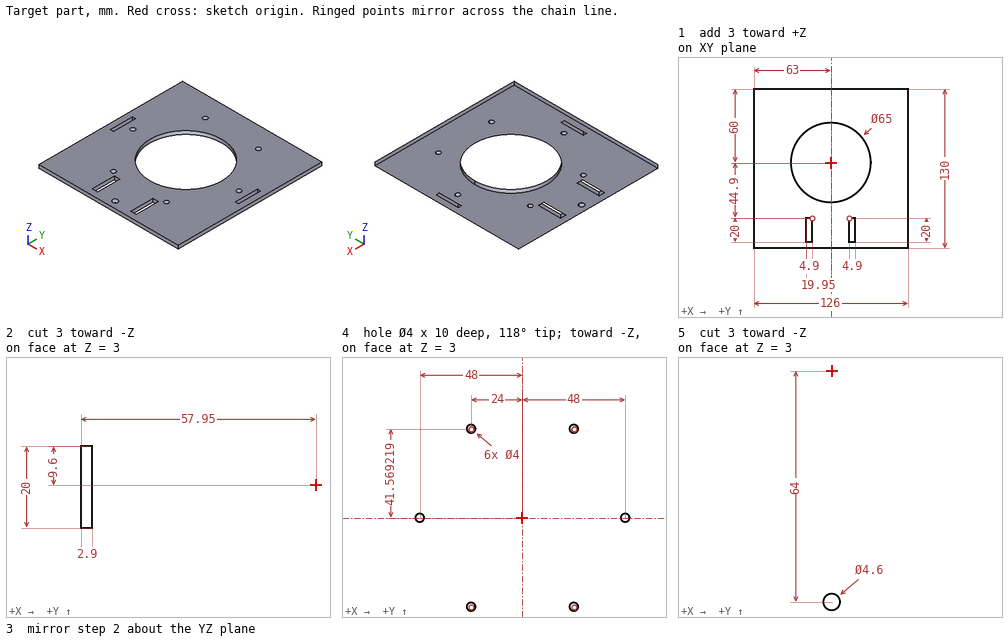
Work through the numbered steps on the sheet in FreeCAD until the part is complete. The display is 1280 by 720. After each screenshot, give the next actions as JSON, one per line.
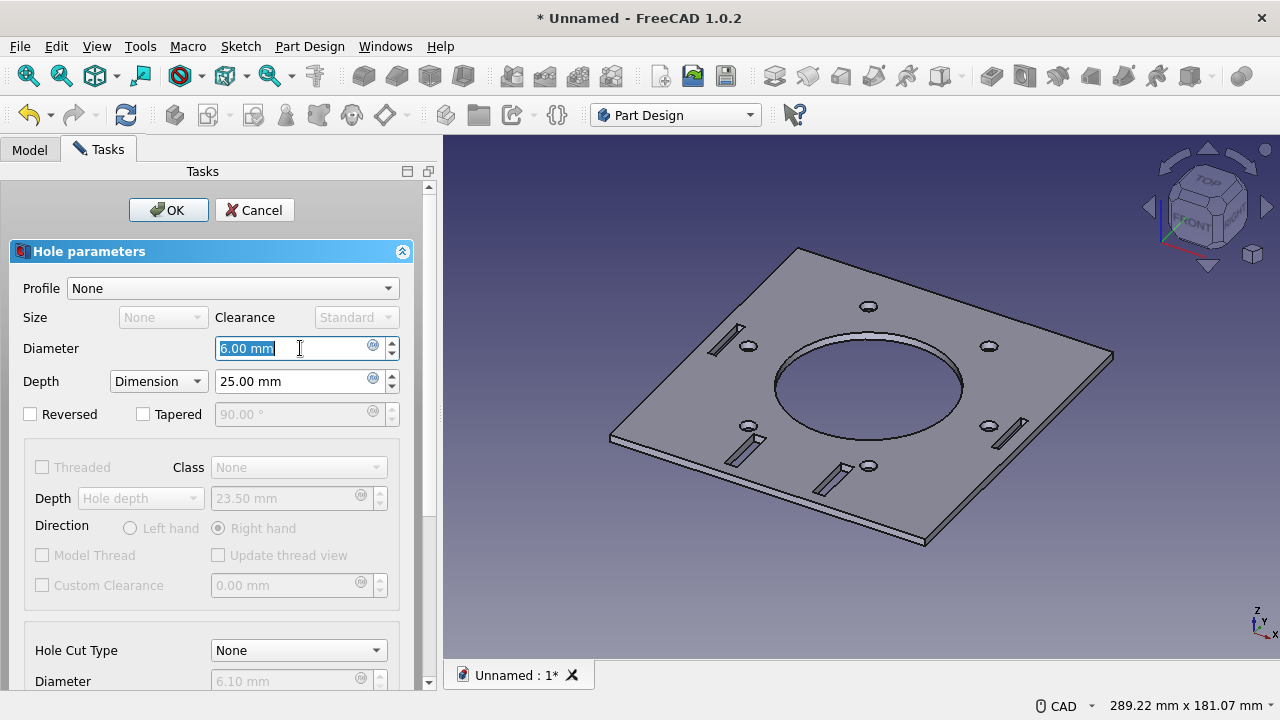
{"action": "type", "text": "4"}
{"action": "key", "text": "Tab"}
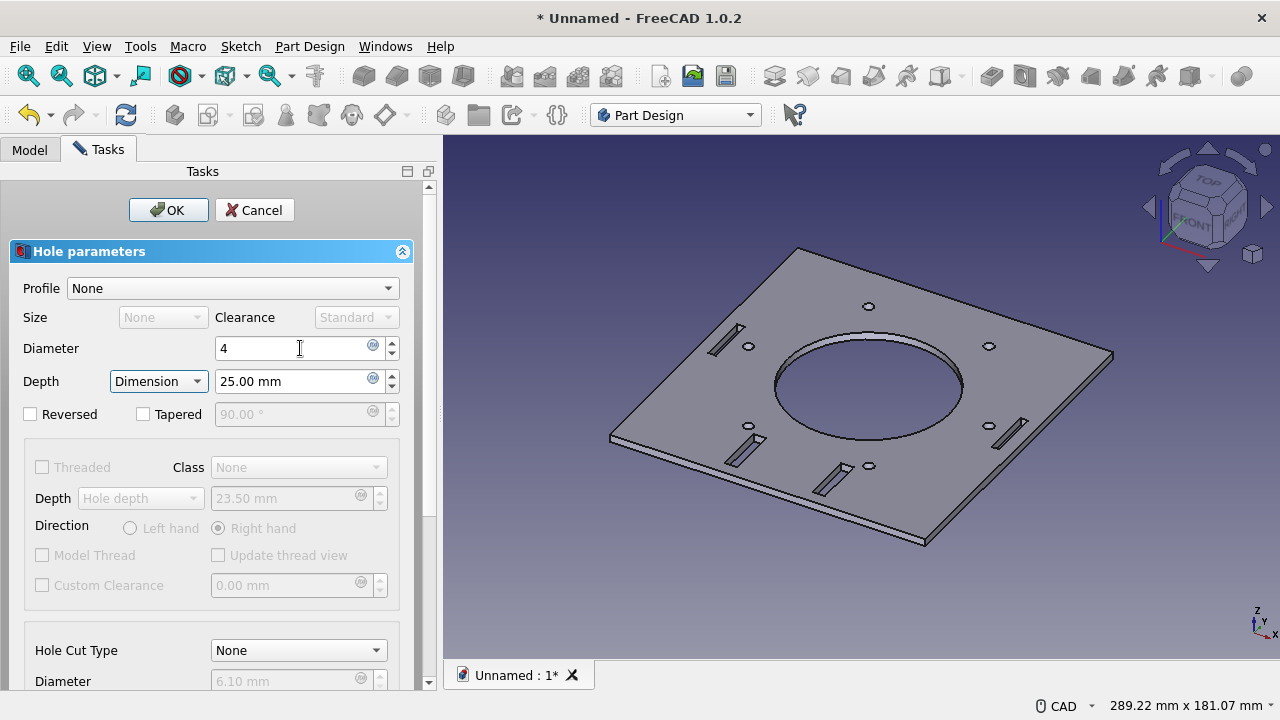
{"action": "triple_click", "coordinate": [300, 382]}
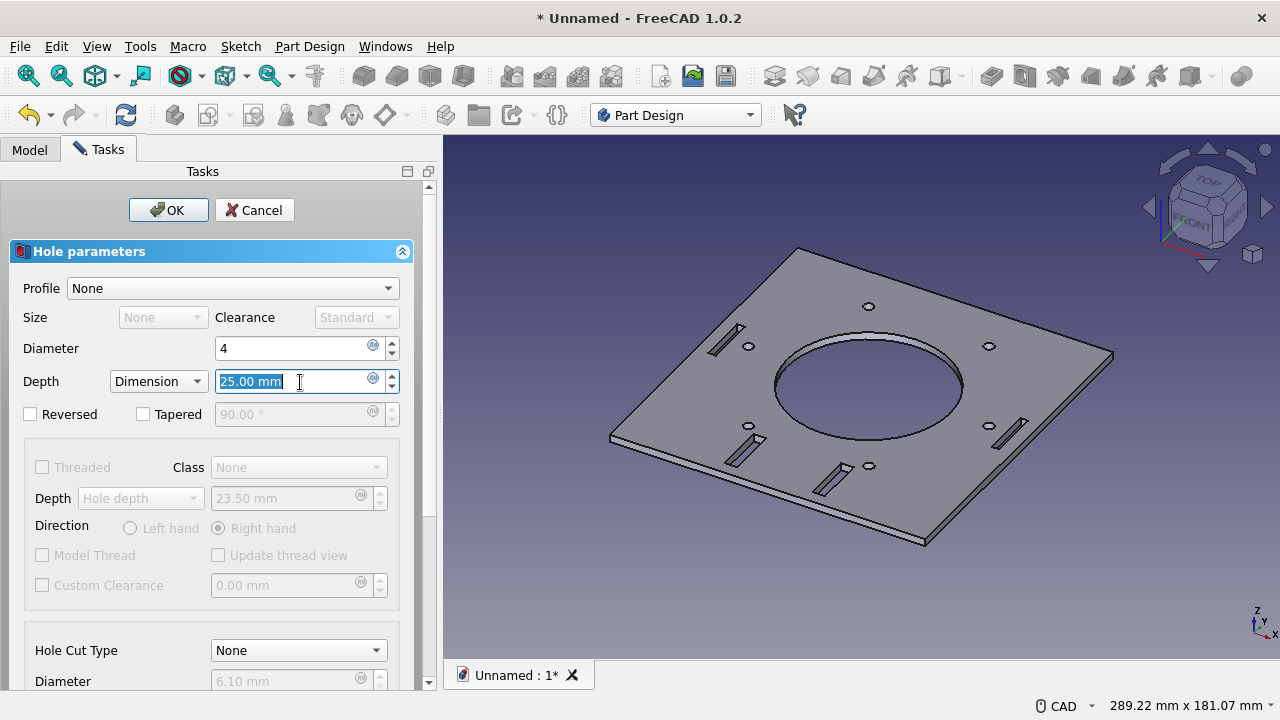
{"action": "type", "text": "10"}
{"action": "key", "text": "Tab"}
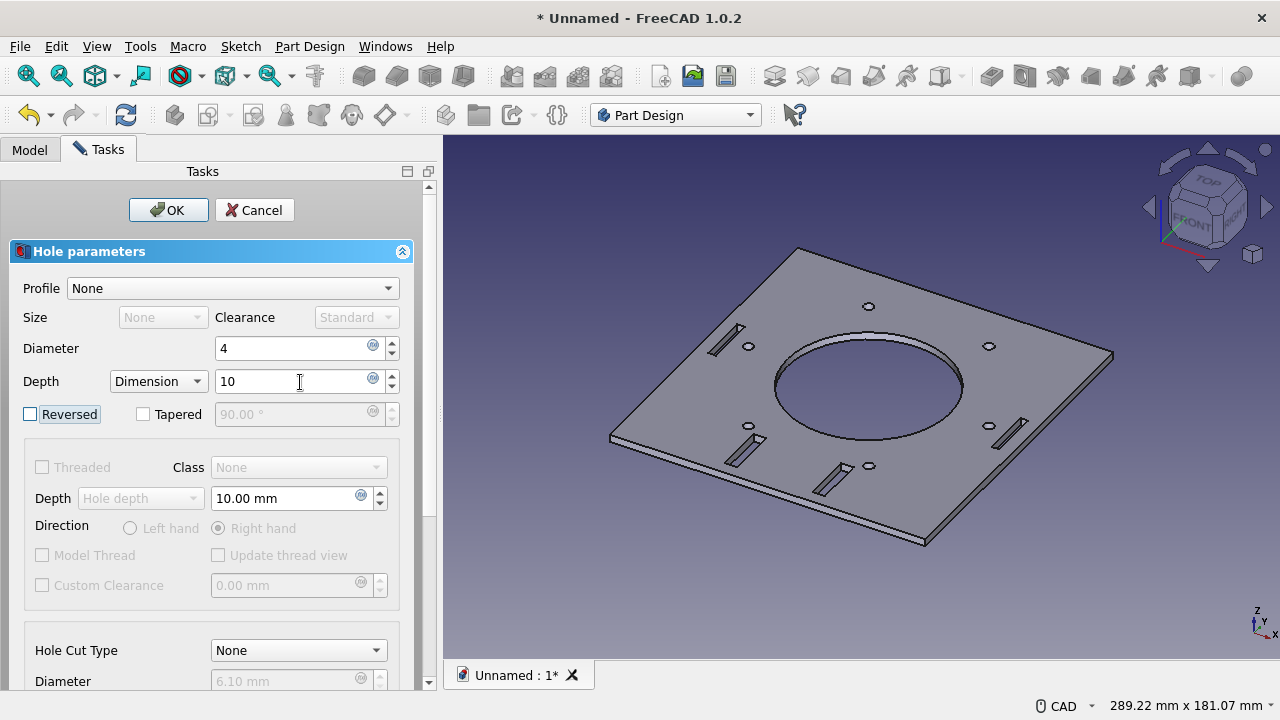
{"action": "left_click", "coordinate": [169, 210]}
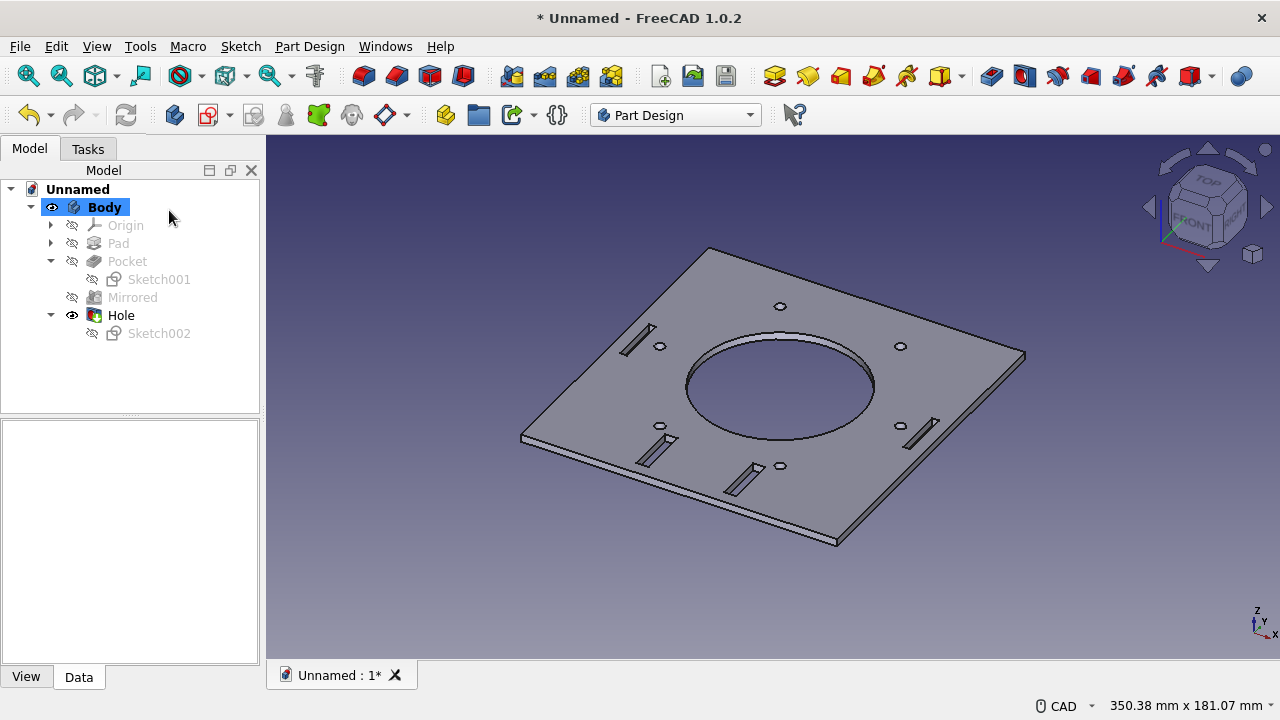
{"action": "left_click", "coordinate": [917, 369]}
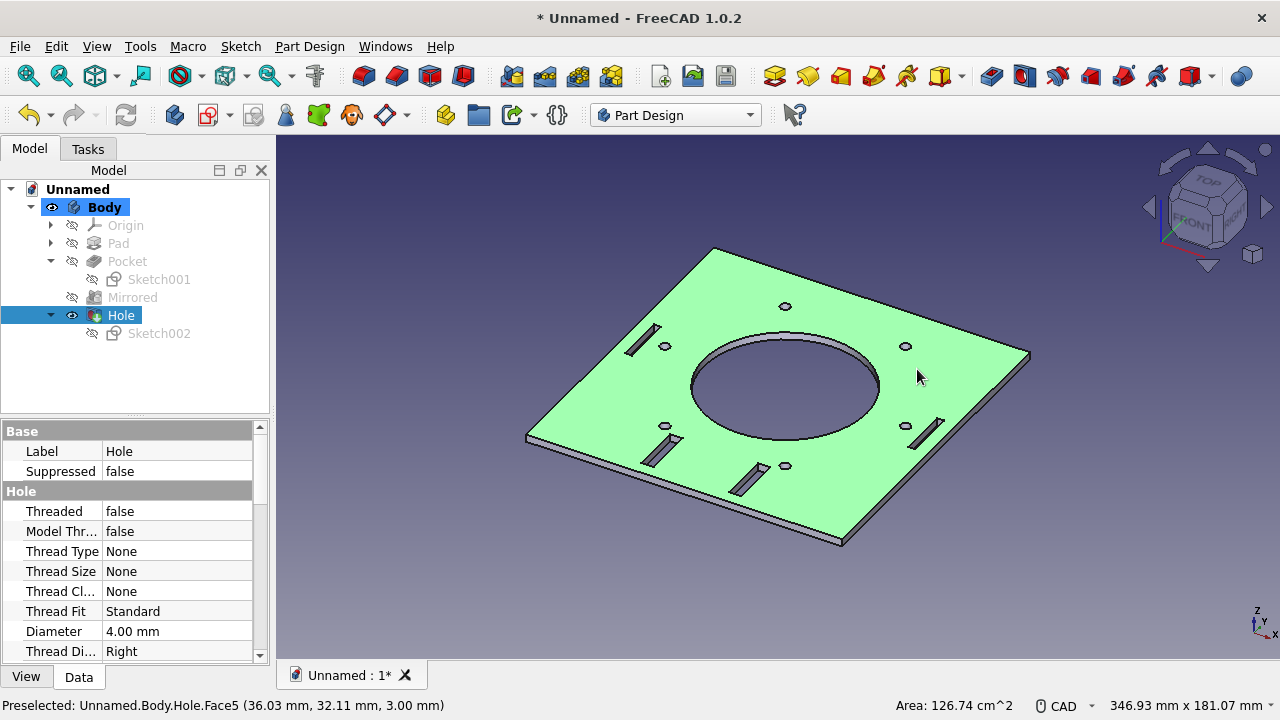
{"action": "left_click", "coordinate": [208, 116]}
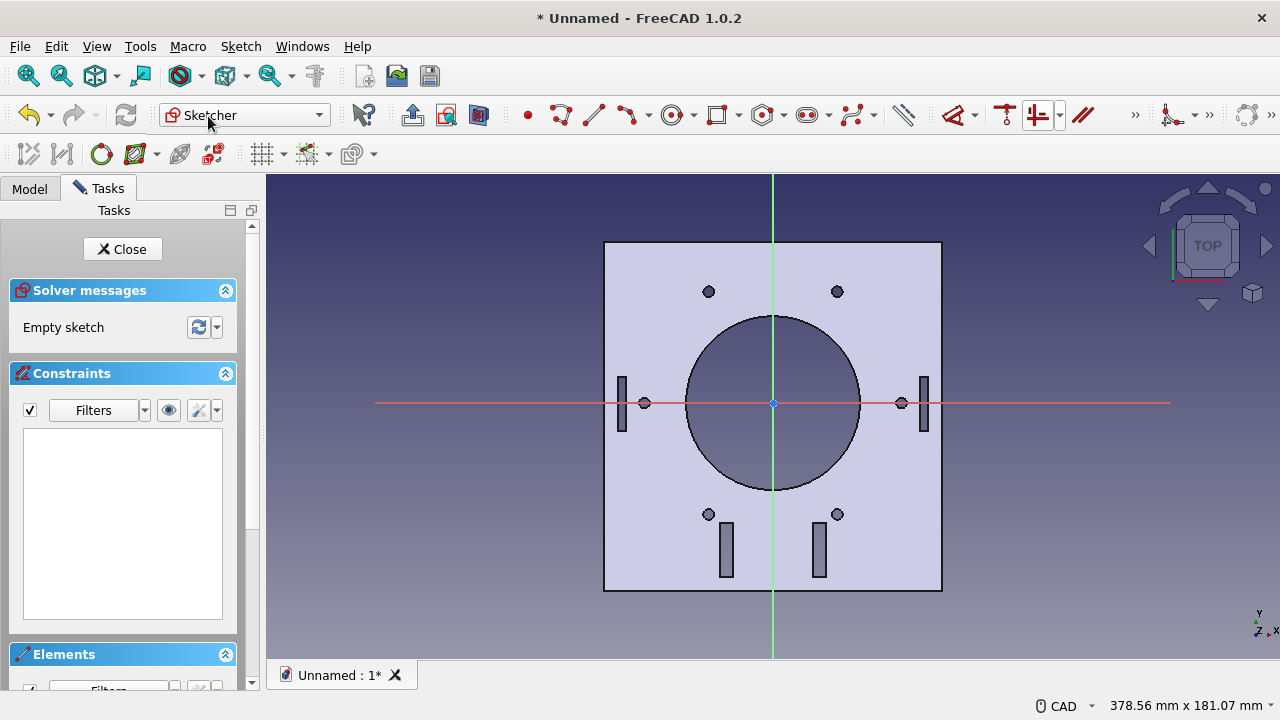
{"action": "scroll", "coordinate": [777, 583], "scroll_direction": "up", "scroll_amount": 15}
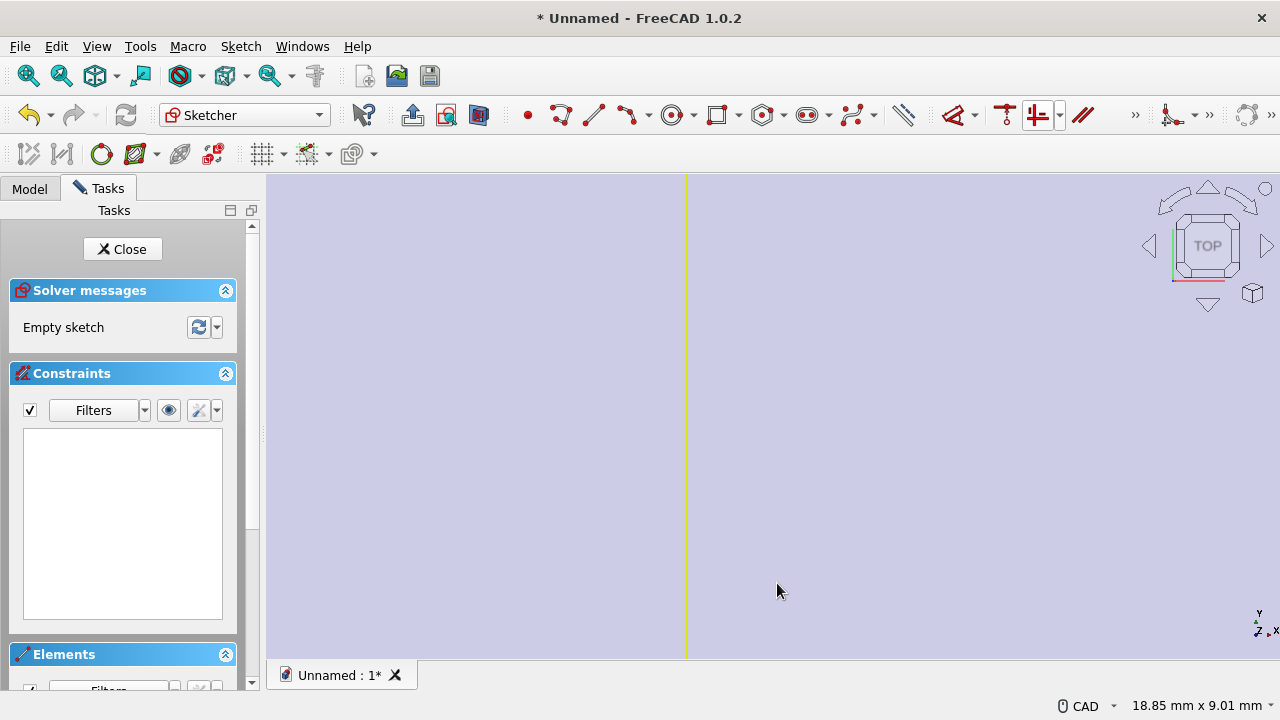
{"action": "left_click", "coordinate": [672, 116]}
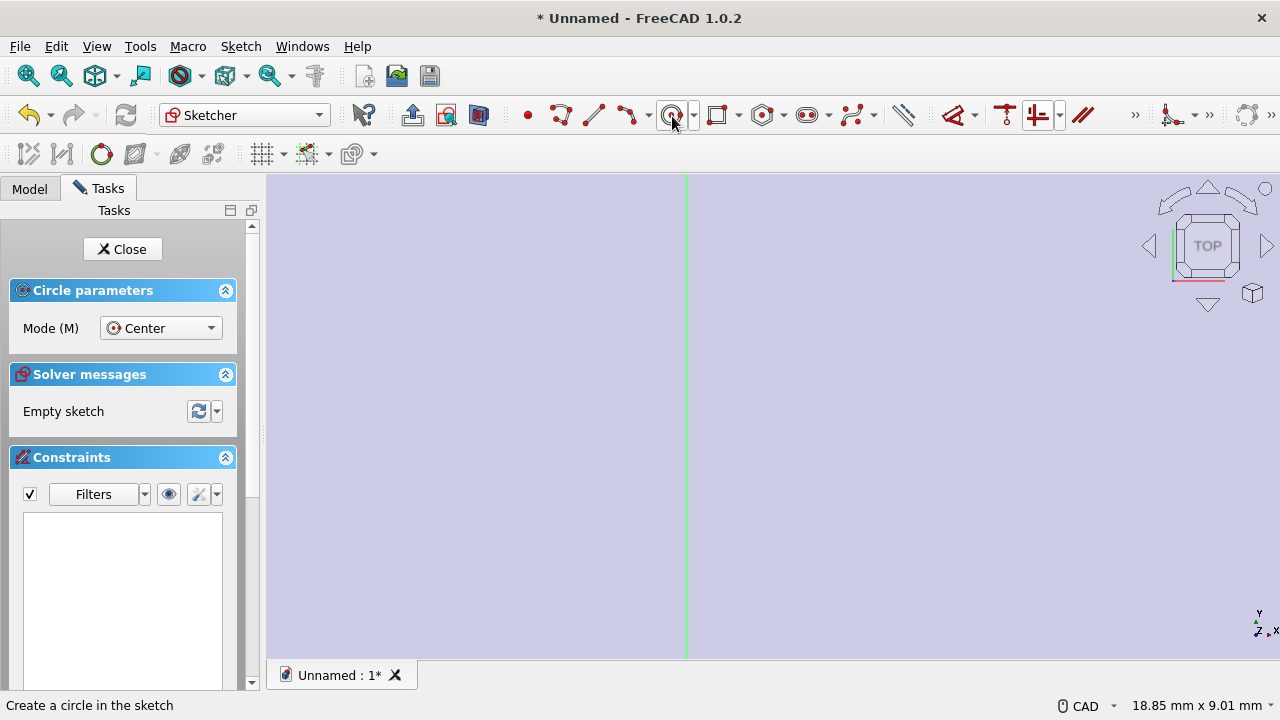
{"action": "left_click", "coordinate": [687, 397]}
{"action": "mouse_move", "coordinate": [775, 309]}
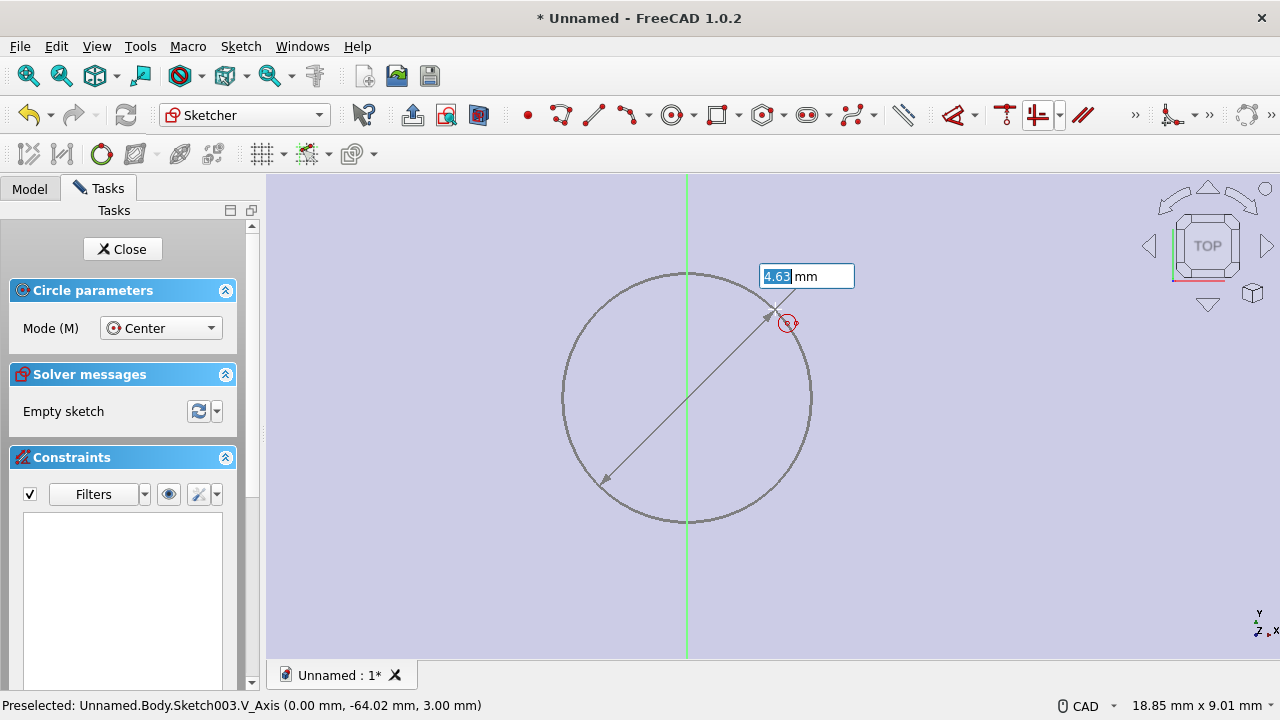
{"action": "type", "text": "4.6"}
{"action": "key", "text": "Return"}
{"action": "key", "text": "Escape"}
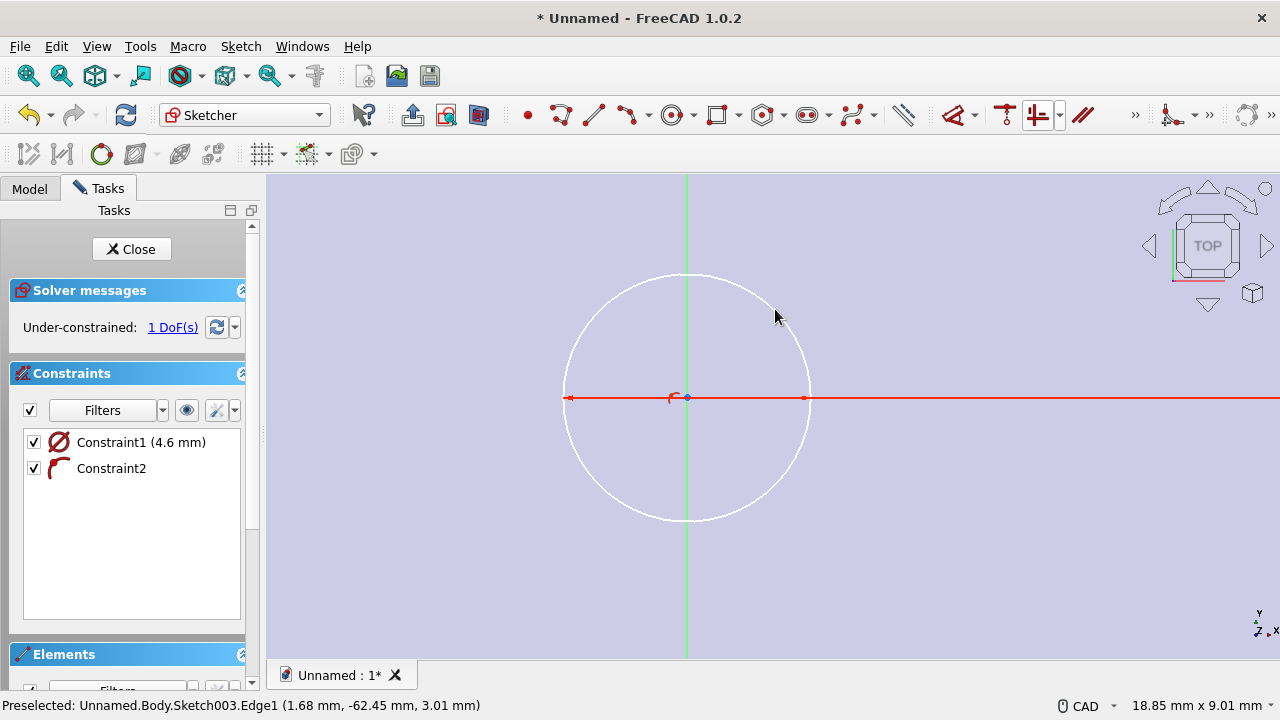
{"action": "left_click", "coordinate": [952, 116]}